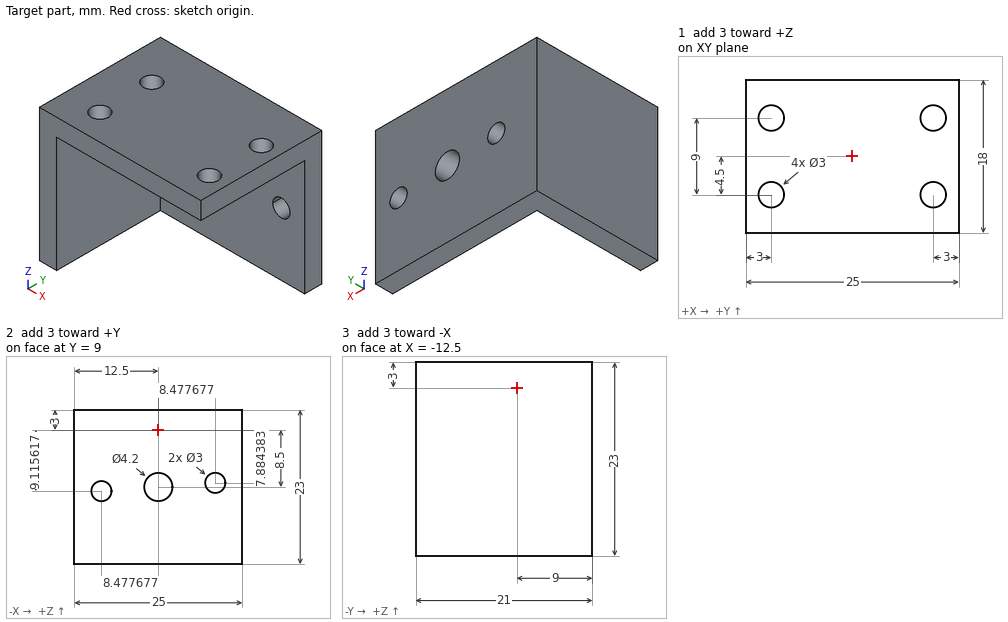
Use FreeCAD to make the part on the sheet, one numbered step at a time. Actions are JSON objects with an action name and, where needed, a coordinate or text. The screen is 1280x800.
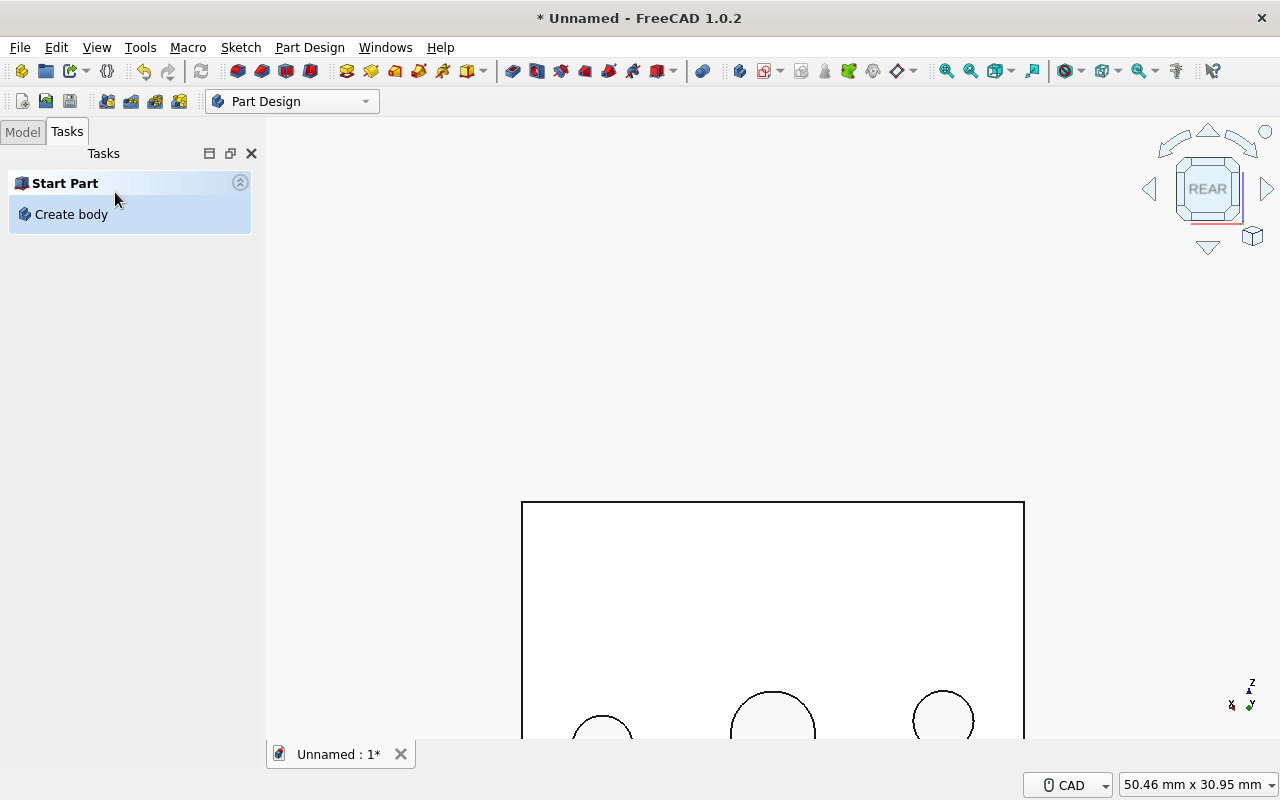
{"action": "key", "text": "v f"}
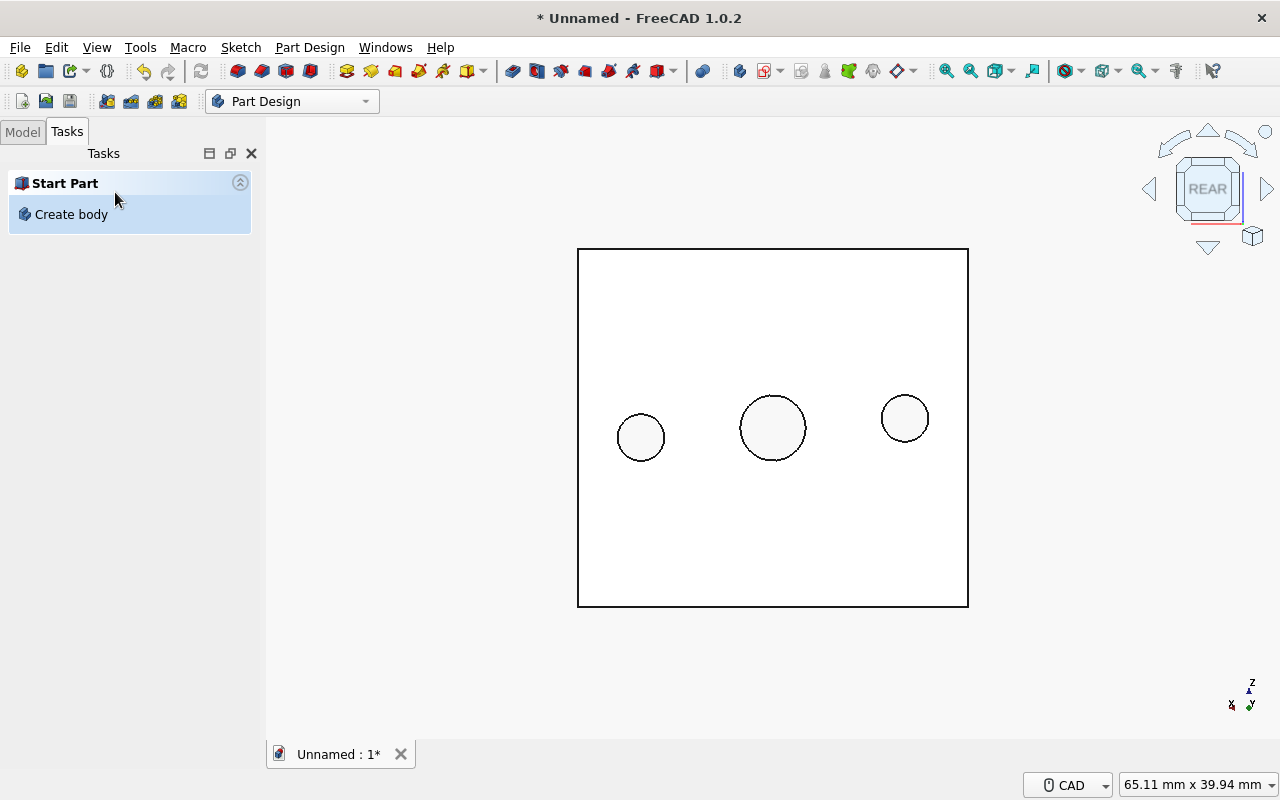
{"action": "key", "text": "6"}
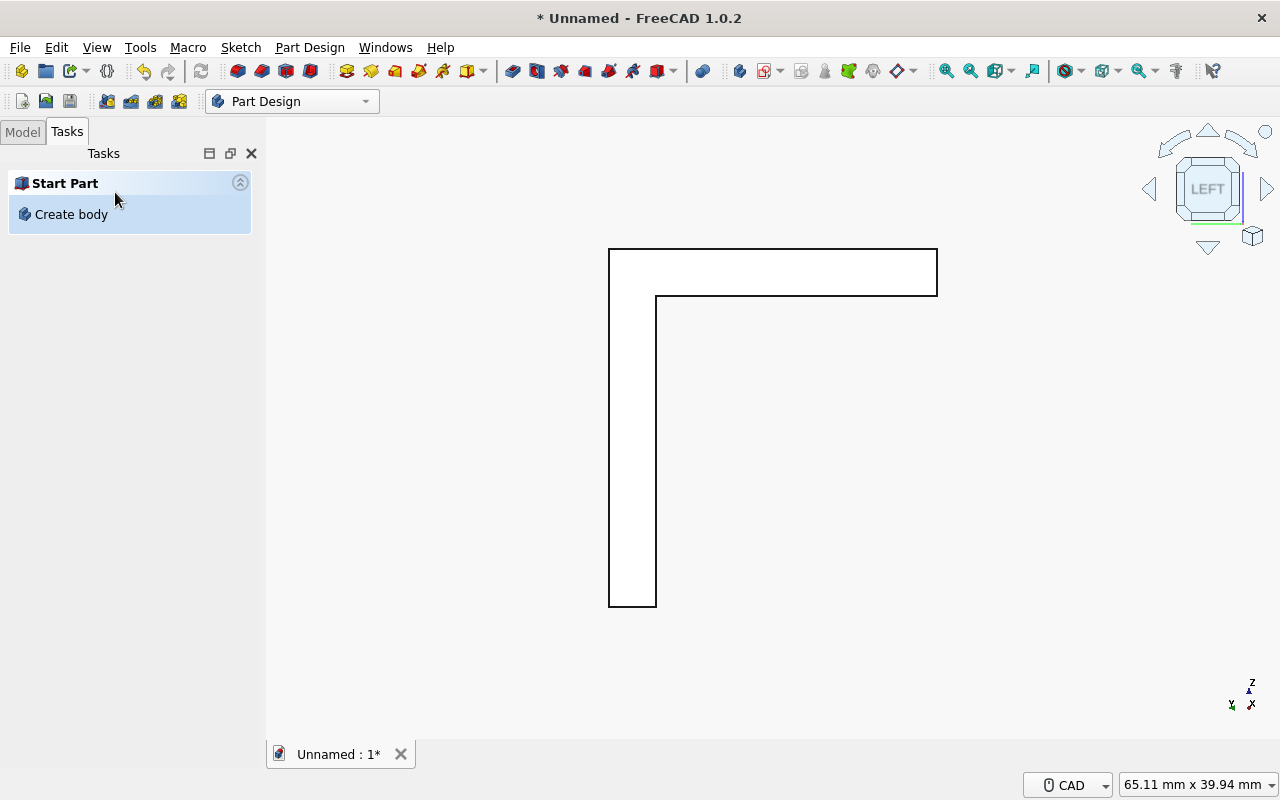
{"action": "left_click", "coordinate": [633, 273]}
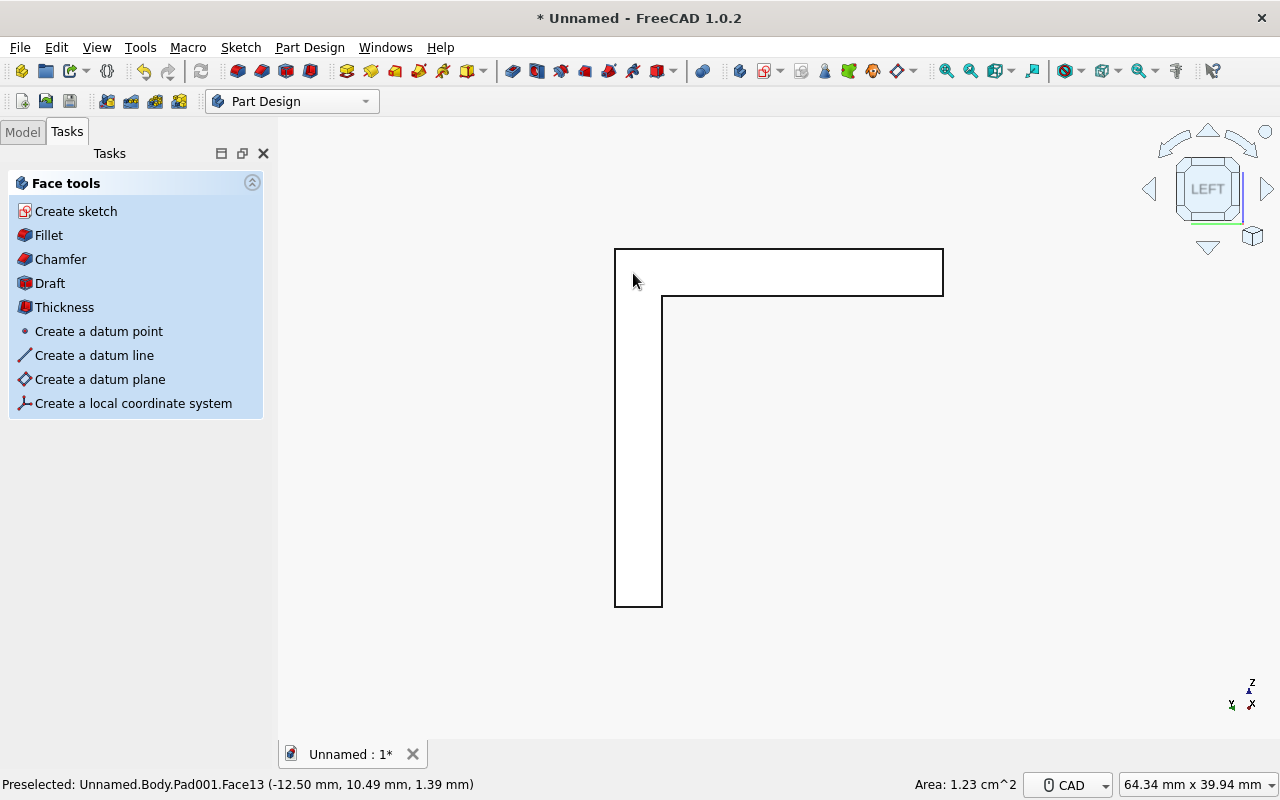
{"action": "left_click", "coordinate": [764, 72]}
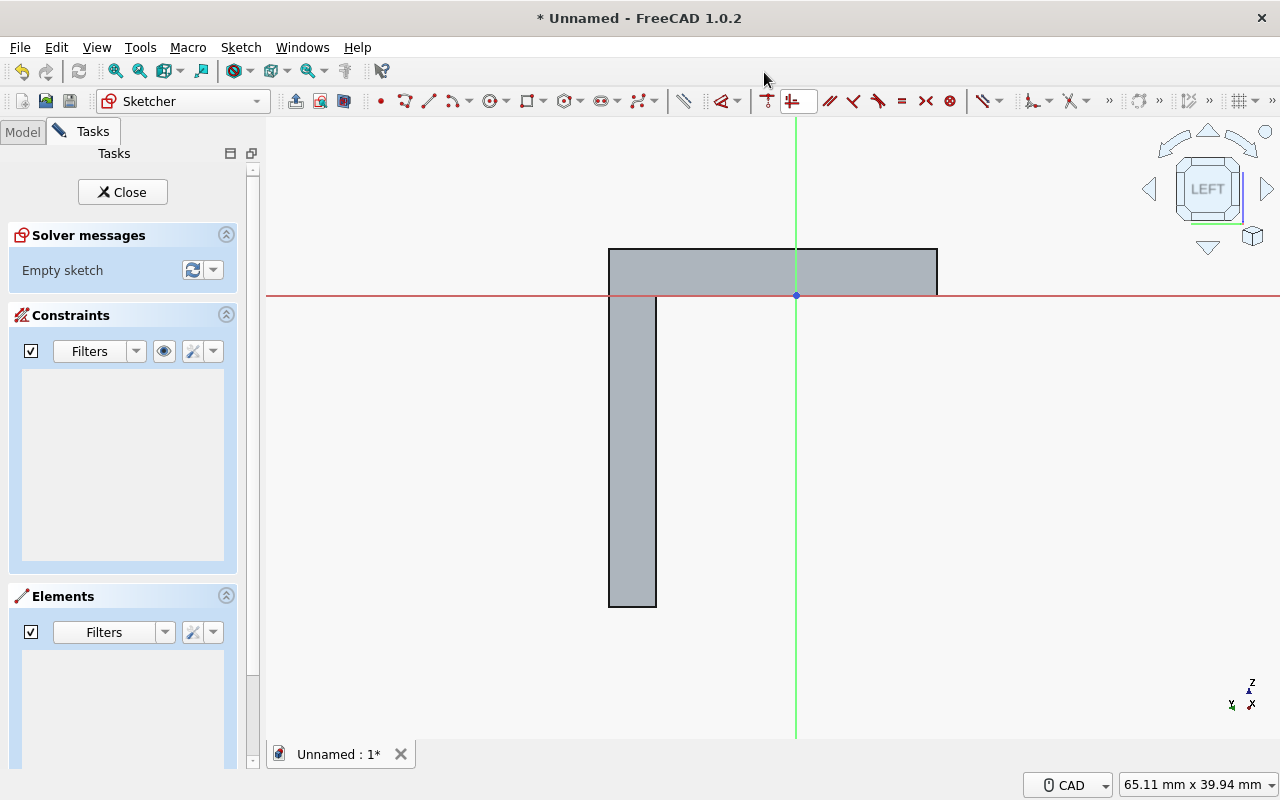
{"action": "left_click", "coordinate": [528, 102]}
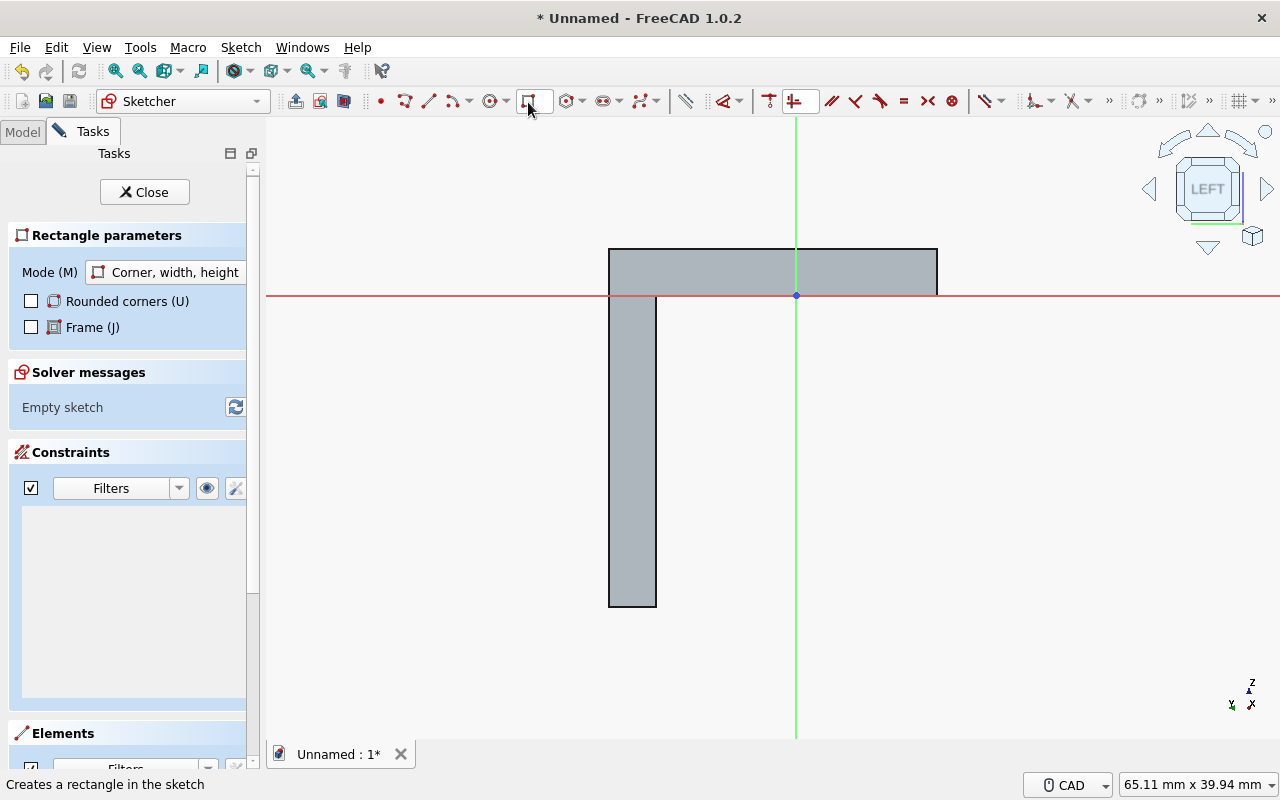
{"action": "left_click", "coordinate": [609, 249]}
{"action": "mouse_move", "coordinate": [937, 607]}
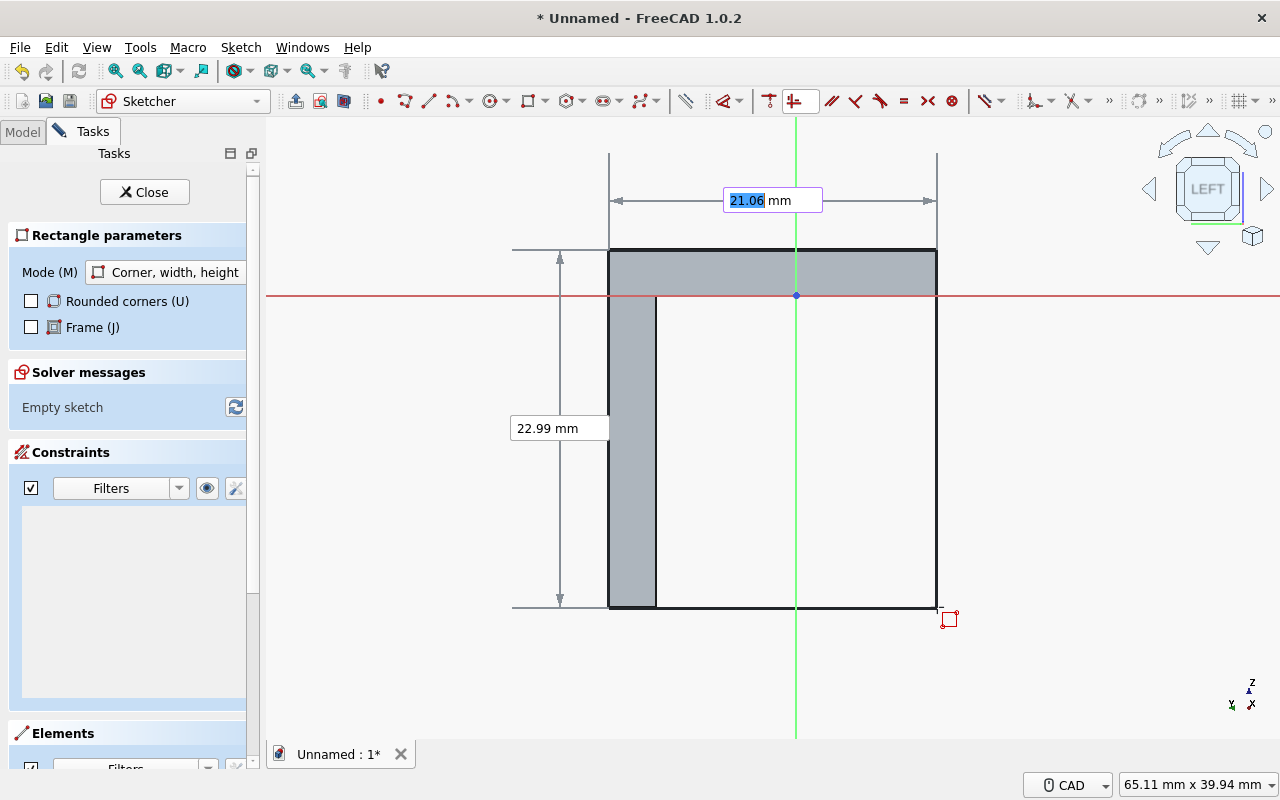
{"action": "type", "text": "21"}
{"action": "key", "text": "Tab"}
{"action": "type", "text": "23"}
{"action": "key", "text": "Return"}
{"action": "key", "text": "Escape"}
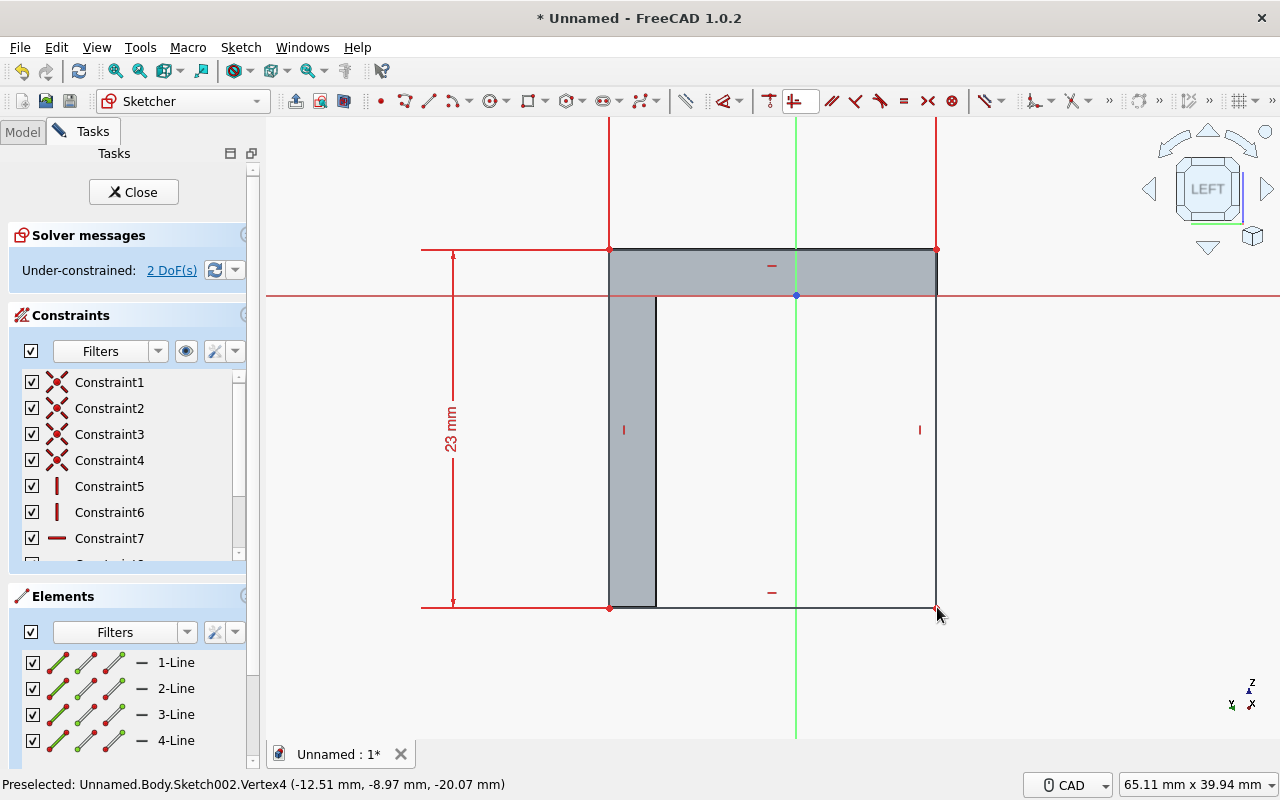
{"action": "key", "text": "d"}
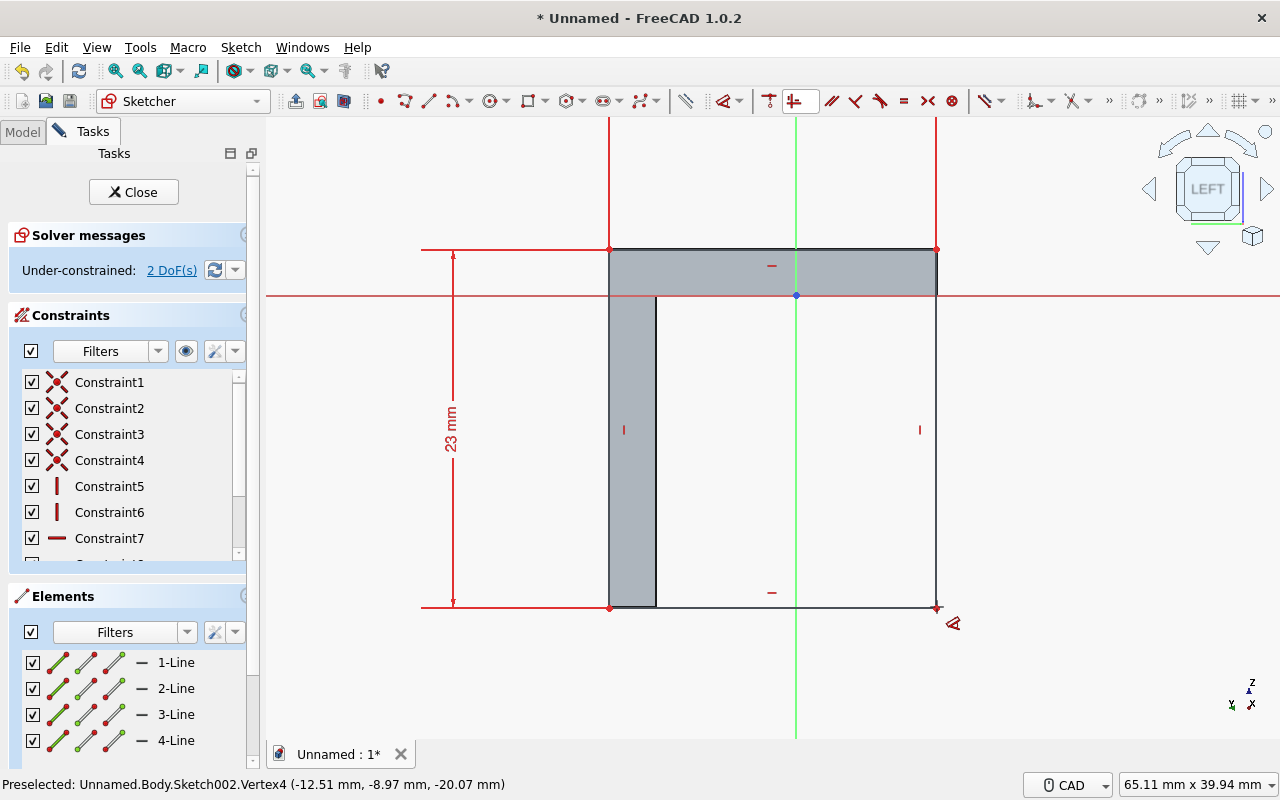
{"action": "left_click", "coordinate": [609, 250]}
{"action": "left_click", "coordinate": [575, 273]}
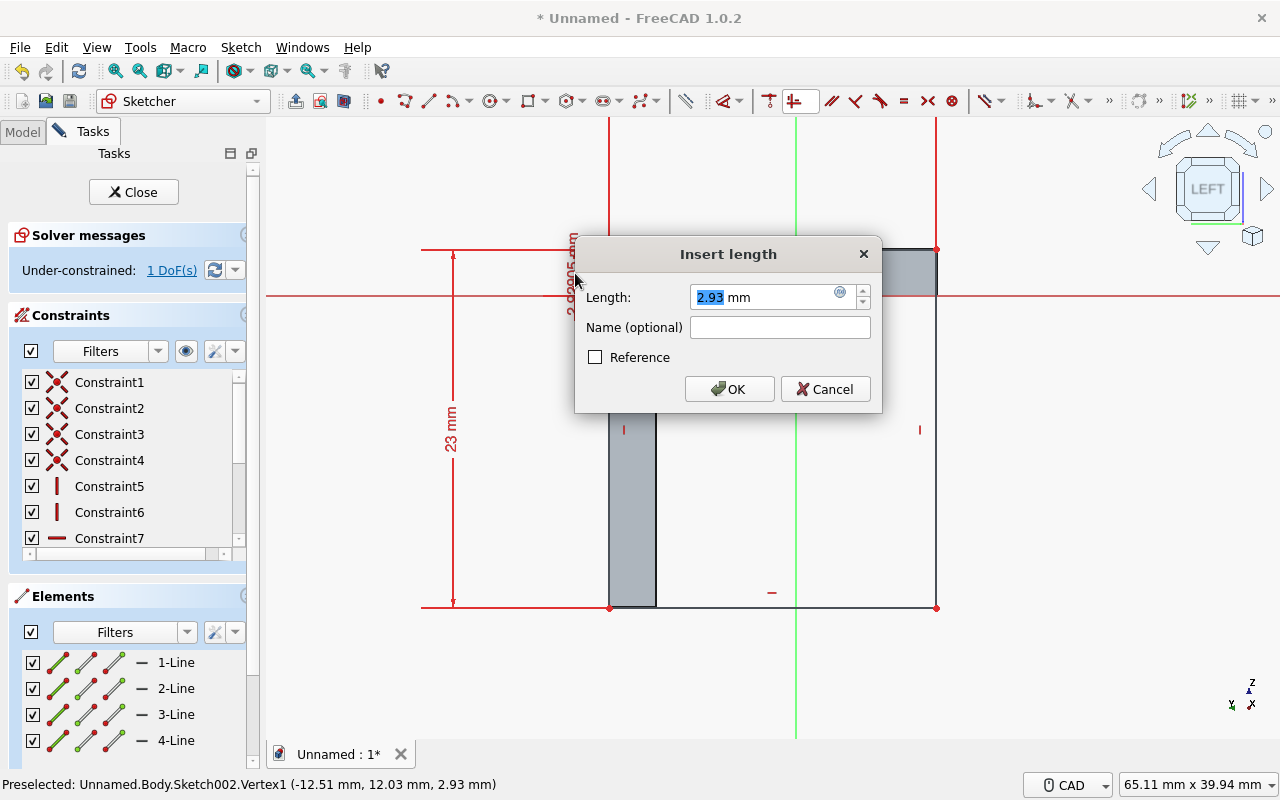
{"action": "type", "text": "3"}
{"action": "key", "text": "Return"}